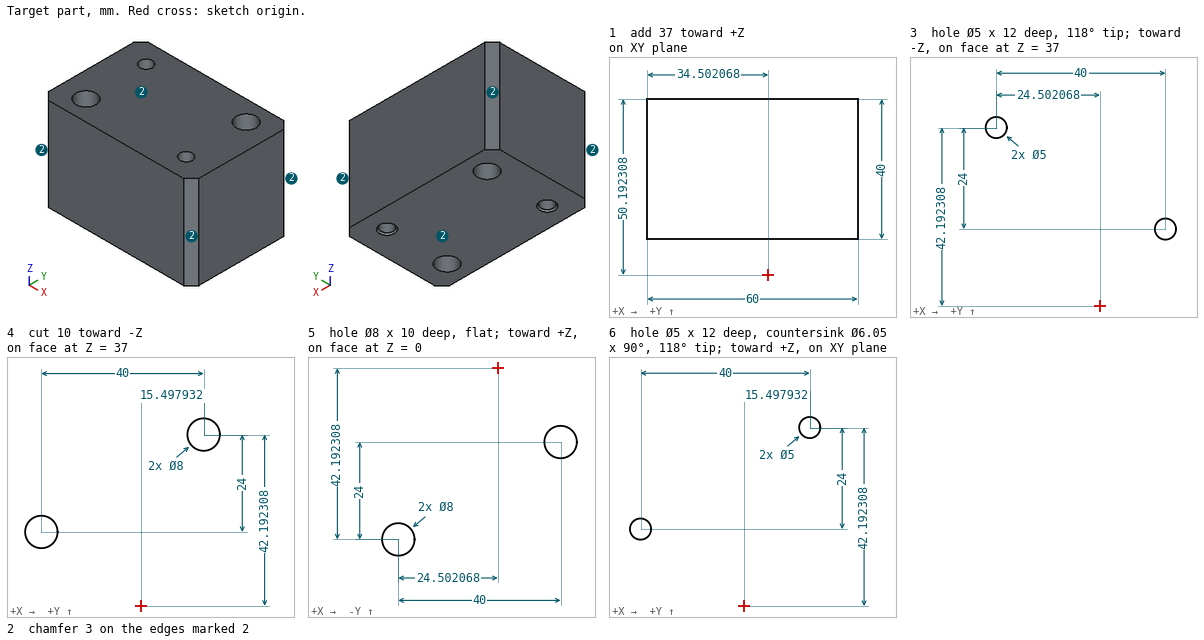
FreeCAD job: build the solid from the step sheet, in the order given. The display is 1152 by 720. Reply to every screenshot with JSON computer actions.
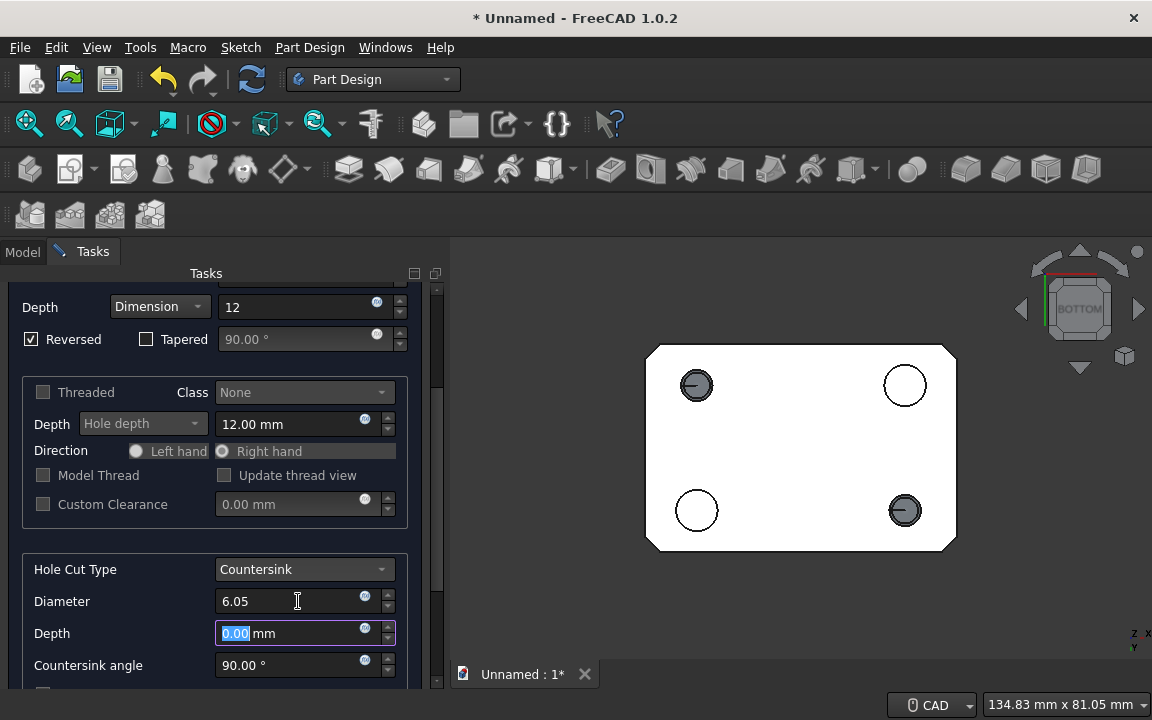
{"action": "scroll", "coordinate": [437, 486], "scroll_direction": "up", "scroll_amount": 4}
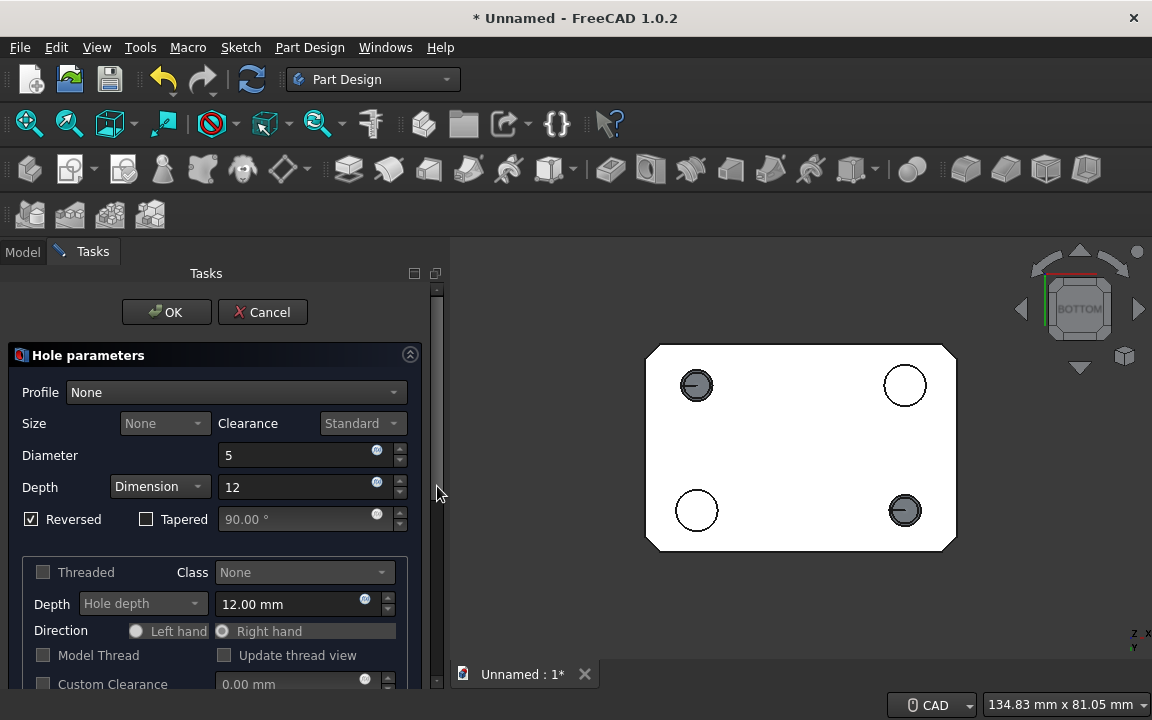
{"action": "left_click", "coordinate": [167, 312]}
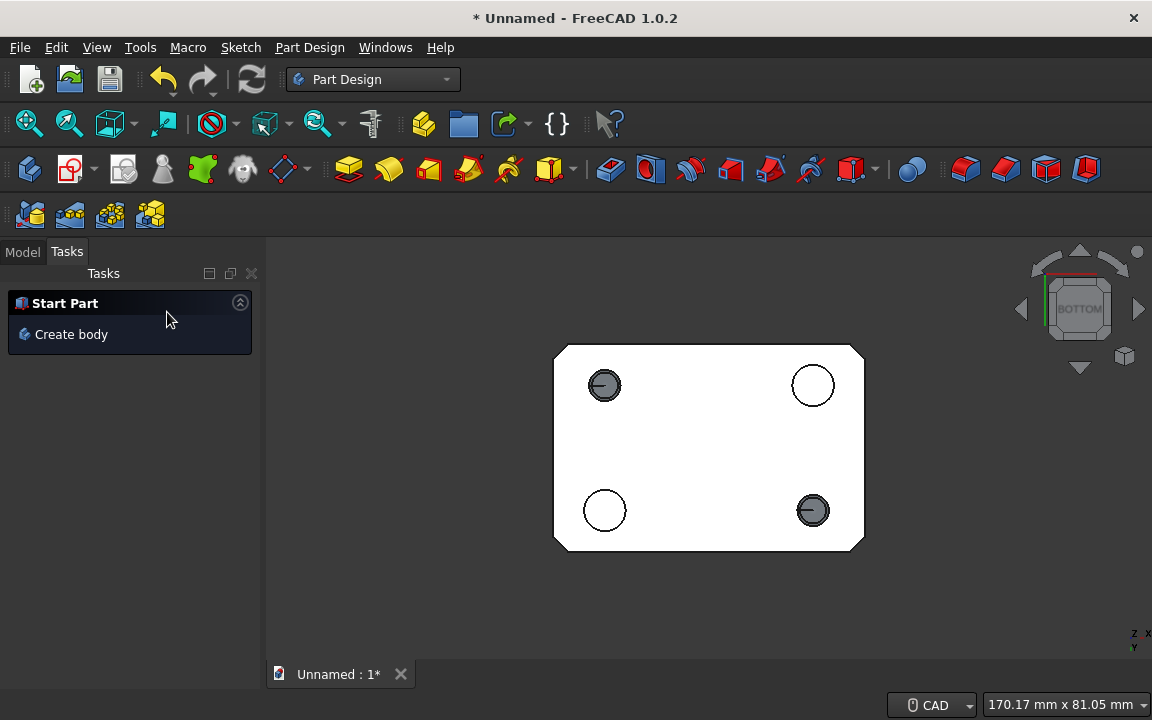
{"action": "key", "text": "0"}